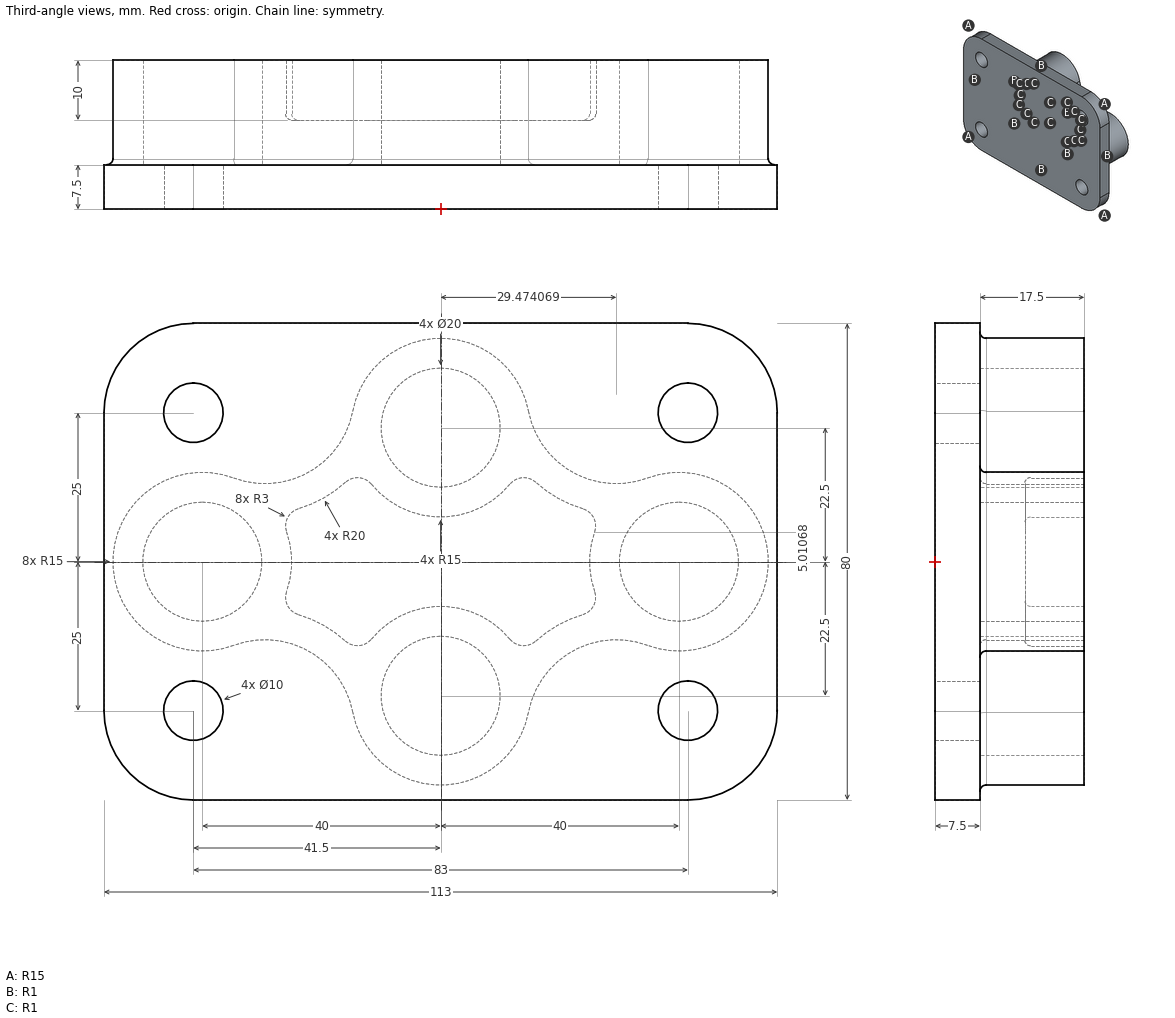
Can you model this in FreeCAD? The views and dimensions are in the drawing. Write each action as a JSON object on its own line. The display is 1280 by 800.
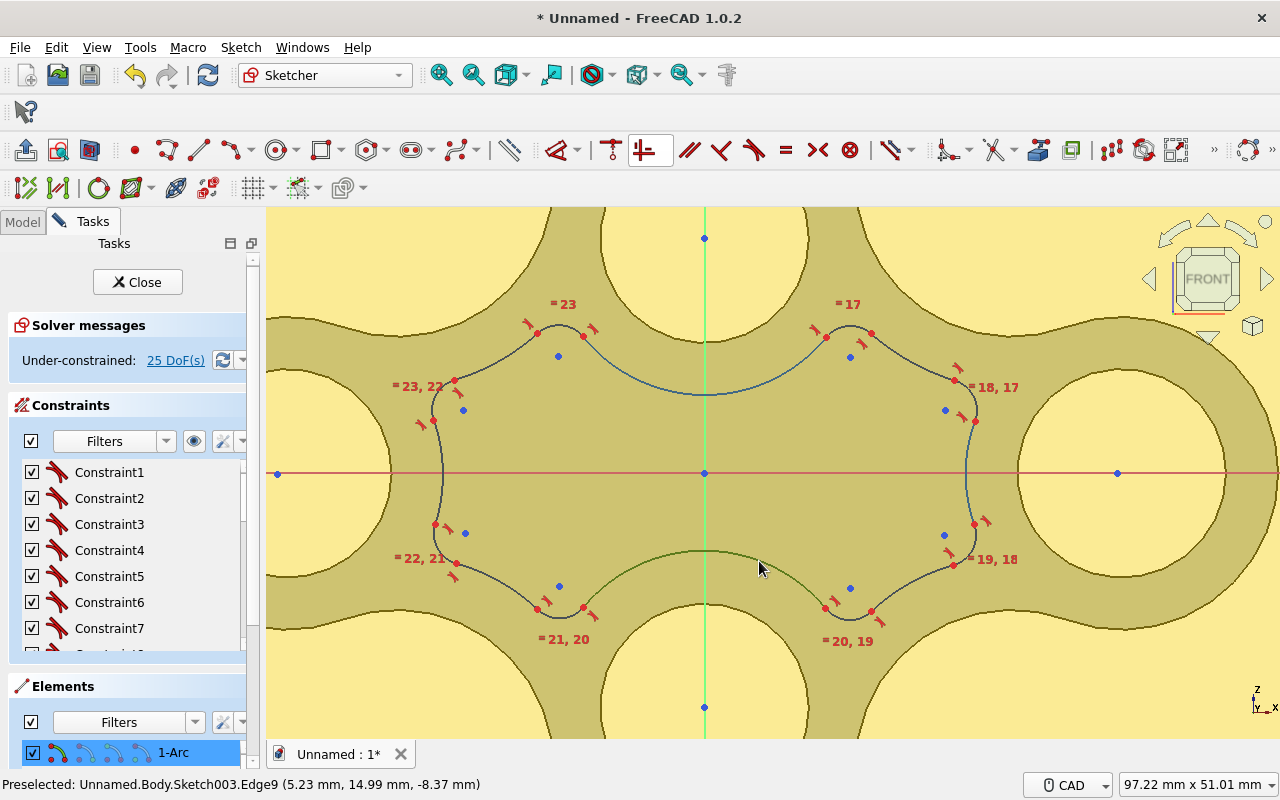
{"action": "left_click", "coordinate": [442, 493]}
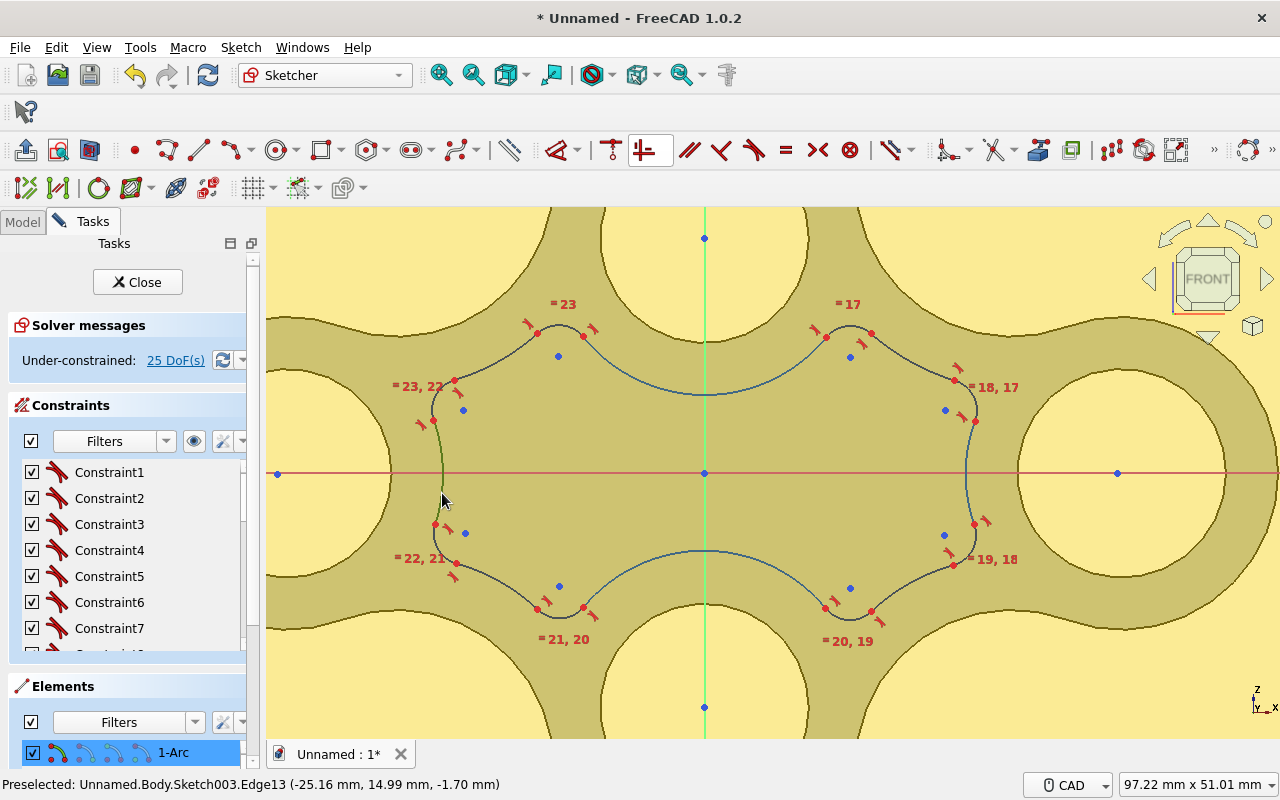
{"action": "key", "text": "e"}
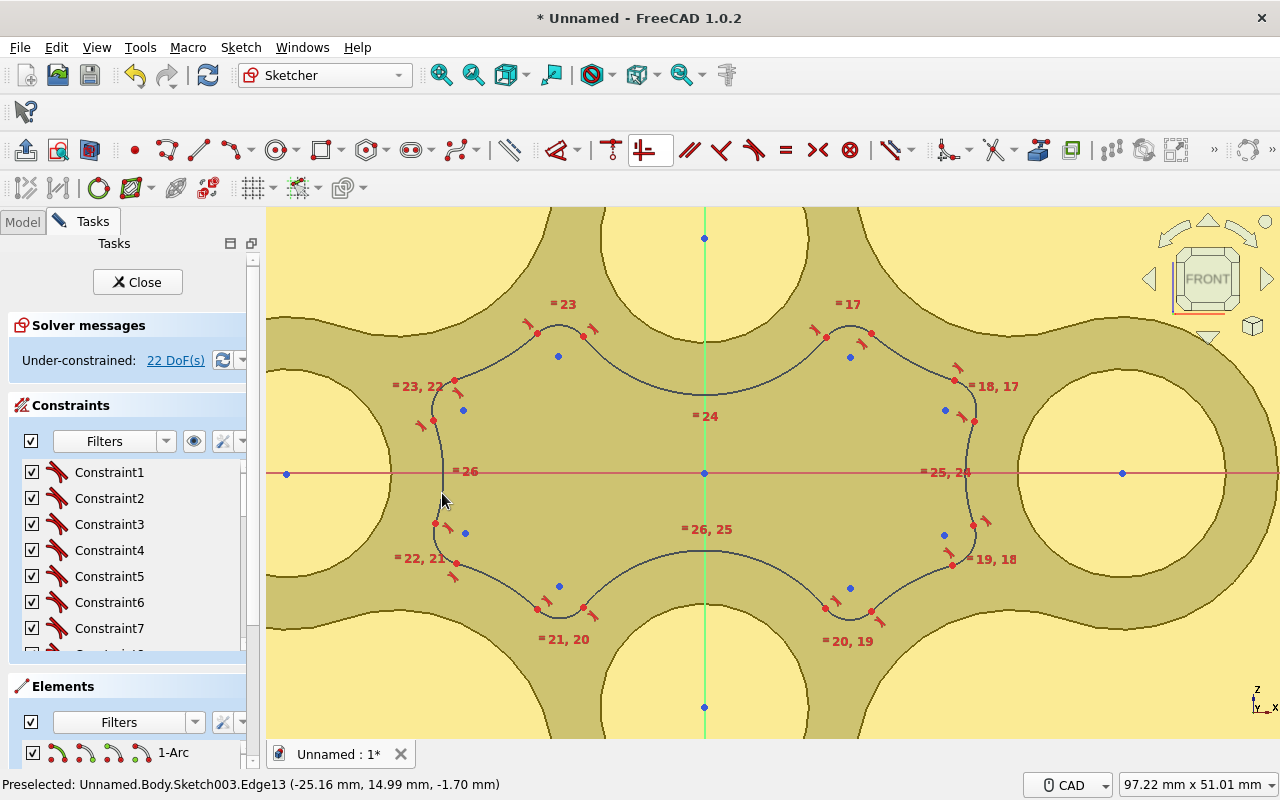
{"action": "left_click", "coordinate": [894, 351]}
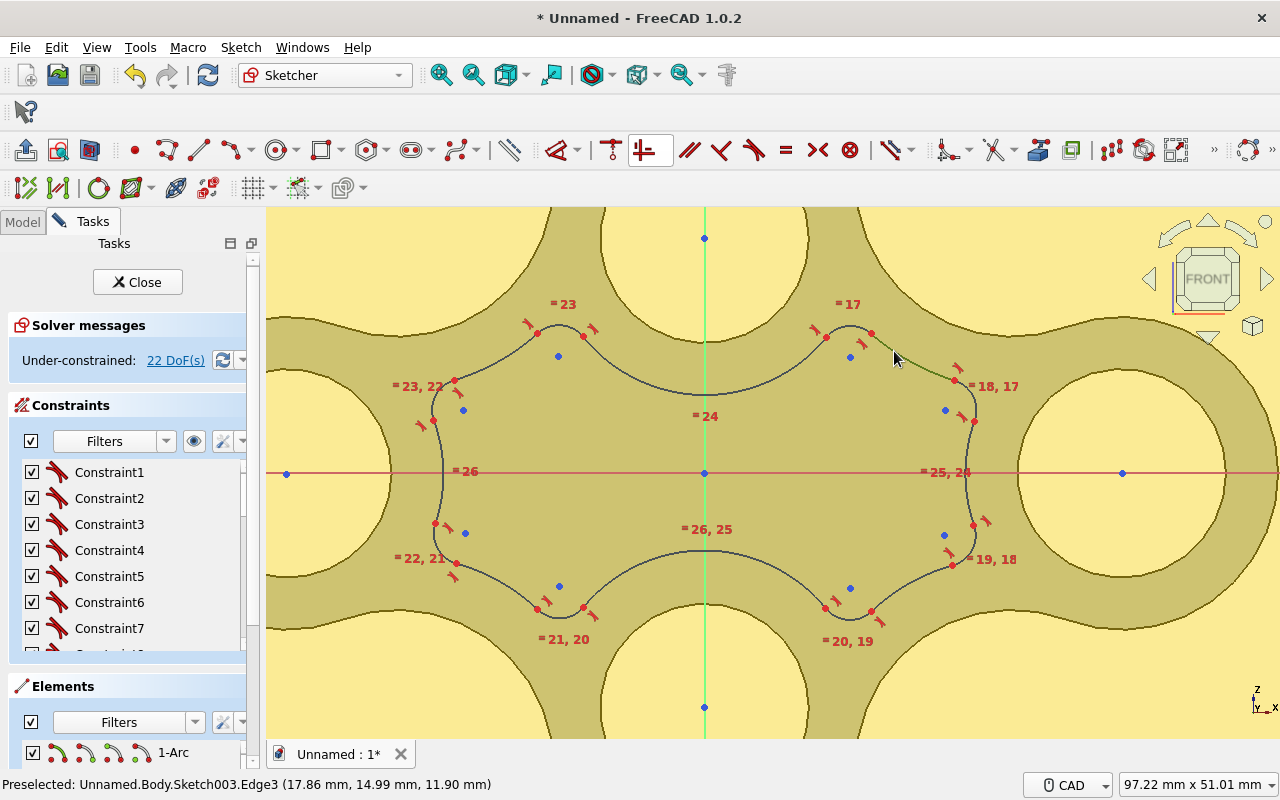
{"action": "left_click", "coordinate": [926, 575]}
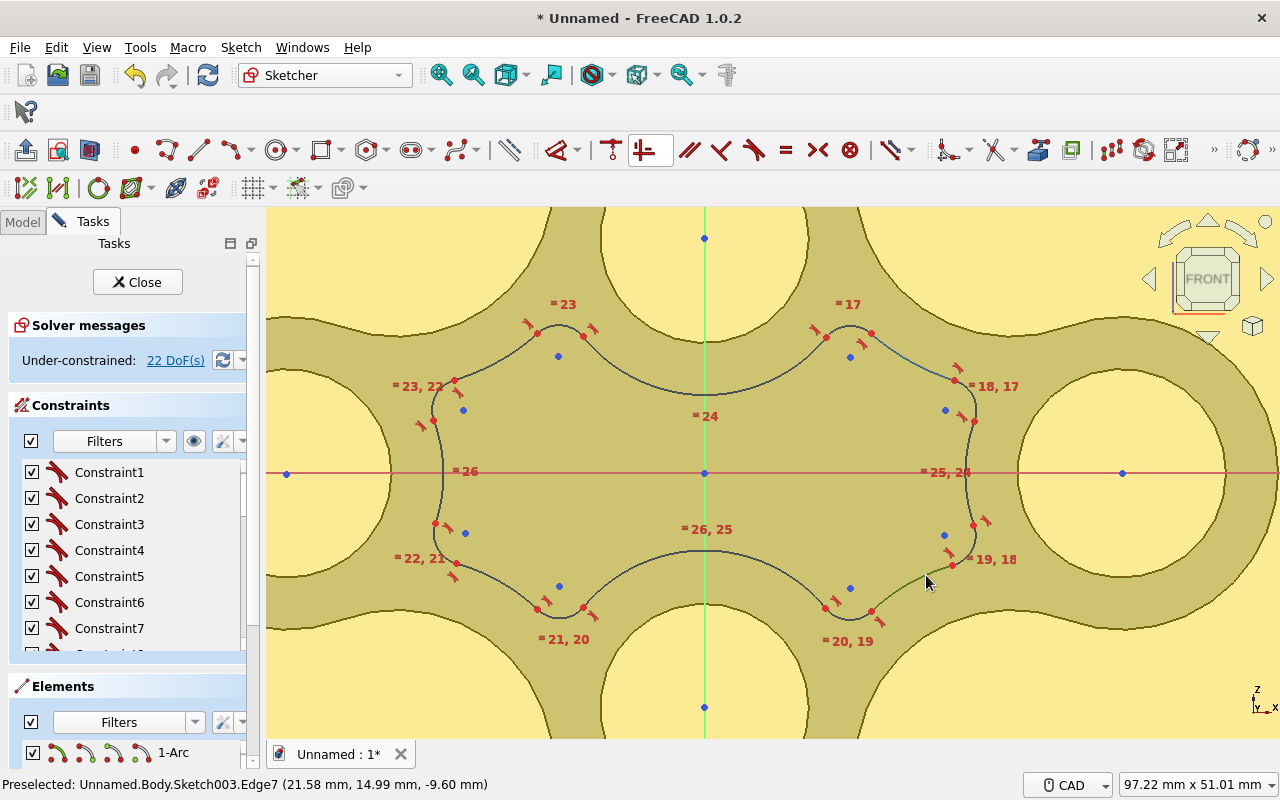
{"action": "left_click", "coordinate": [516, 592]}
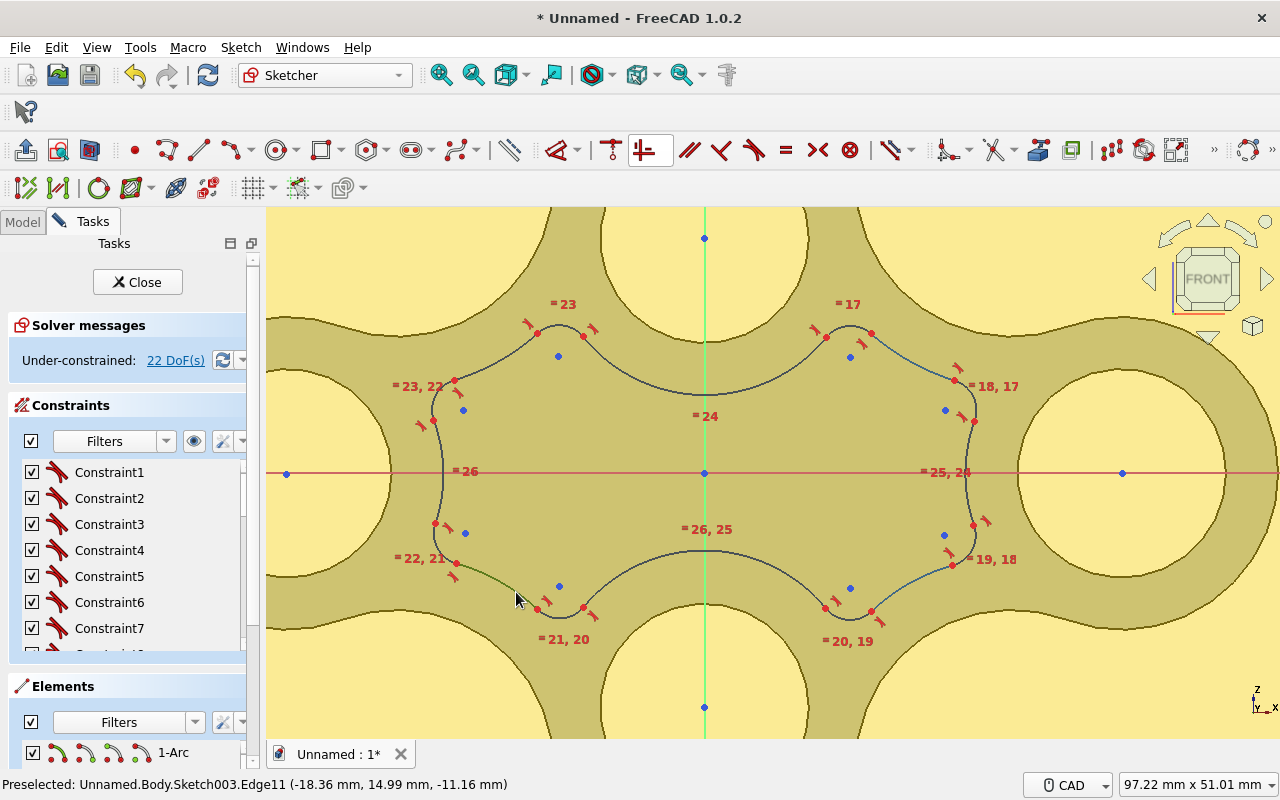
{"action": "left_click", "coordinate": [482, 370]}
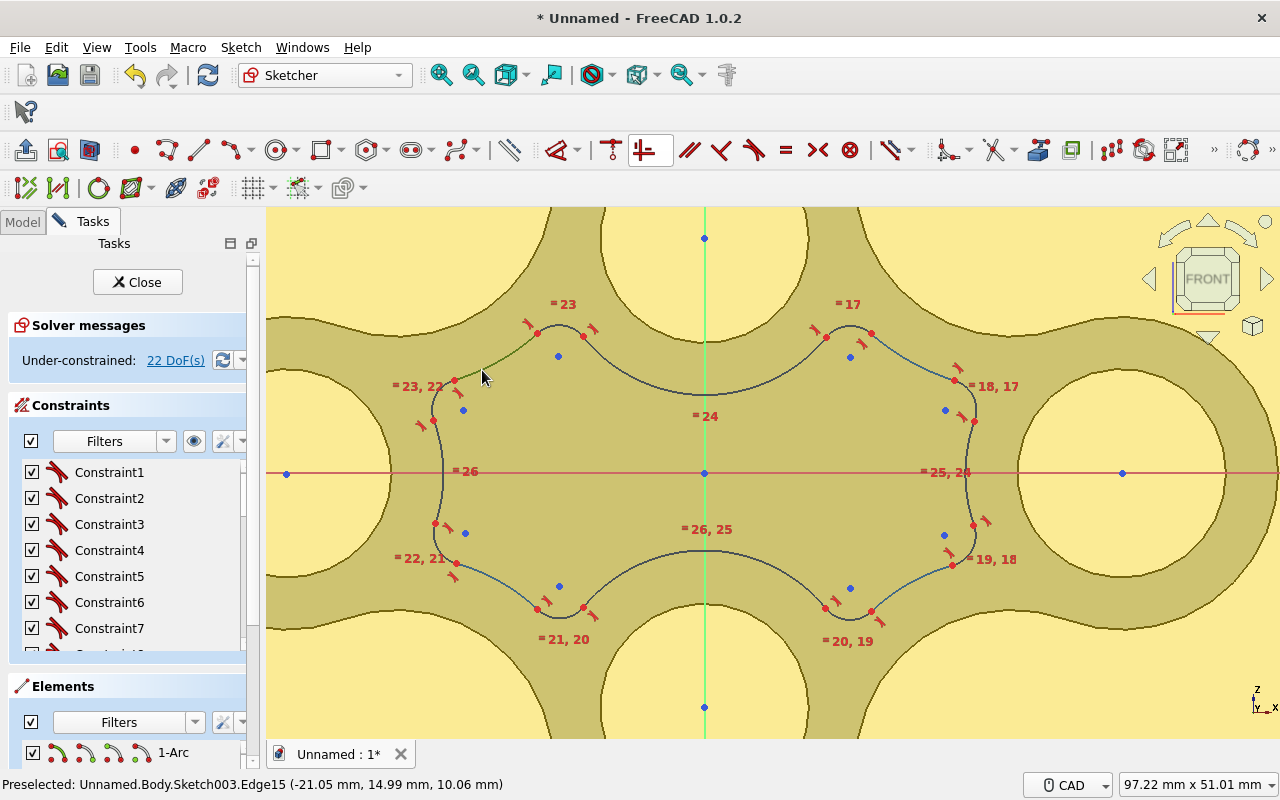
{"action": "key", "text": "e"}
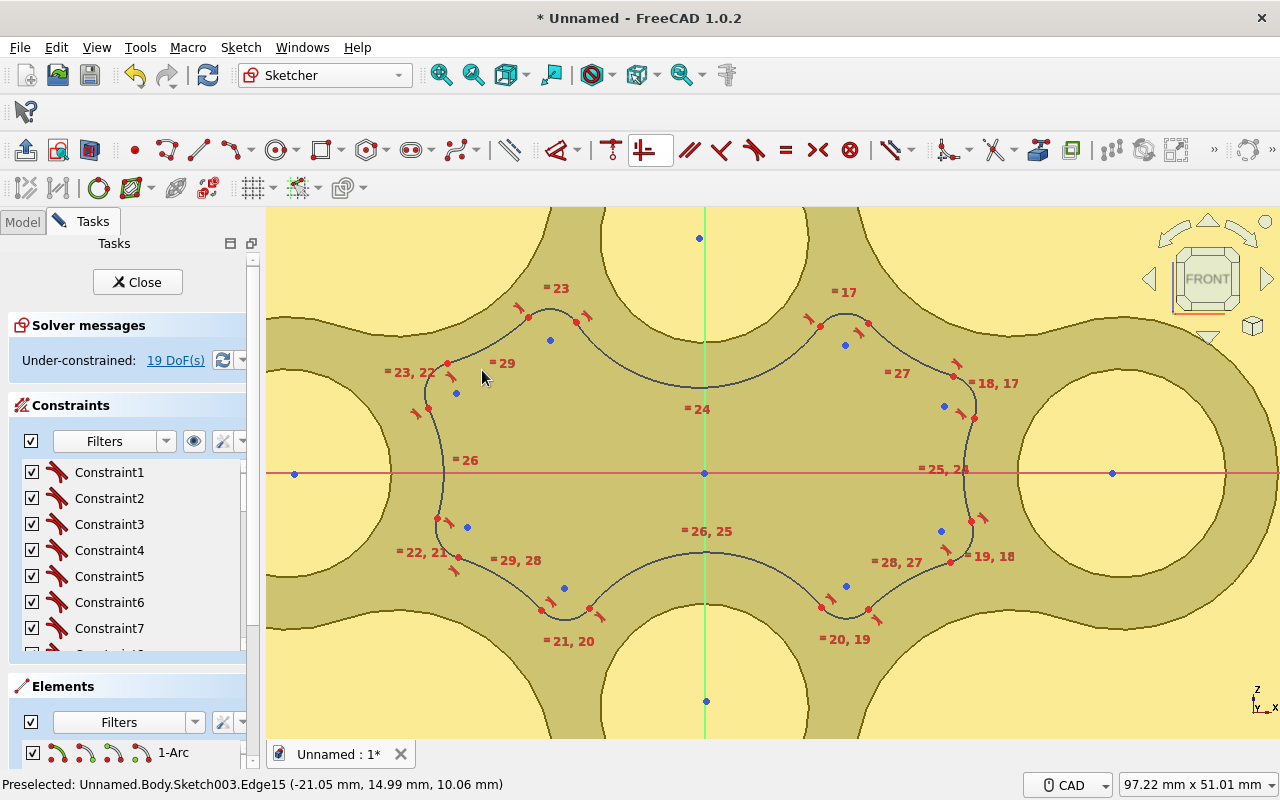
{"action": "left_click", "coordinate": [699, 238]}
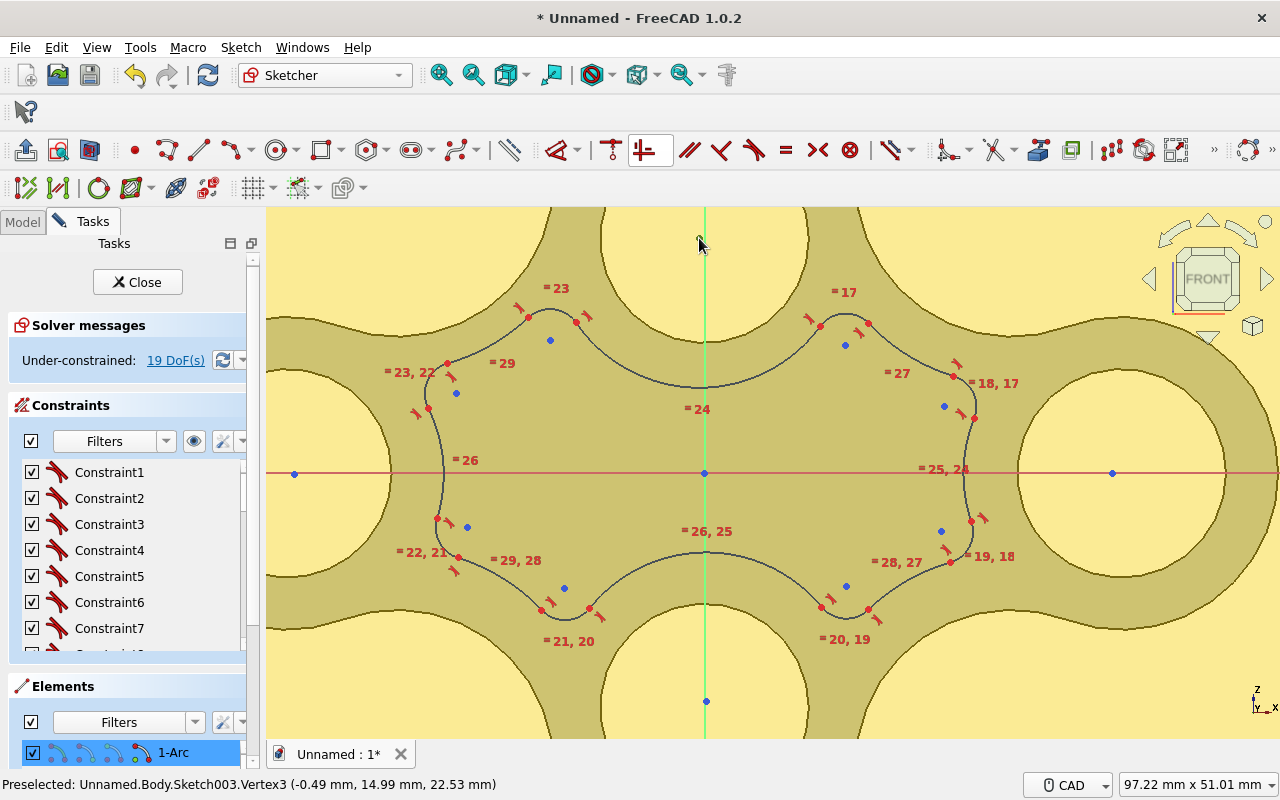
{"action": "left_click", "coordinate": [705, 677]}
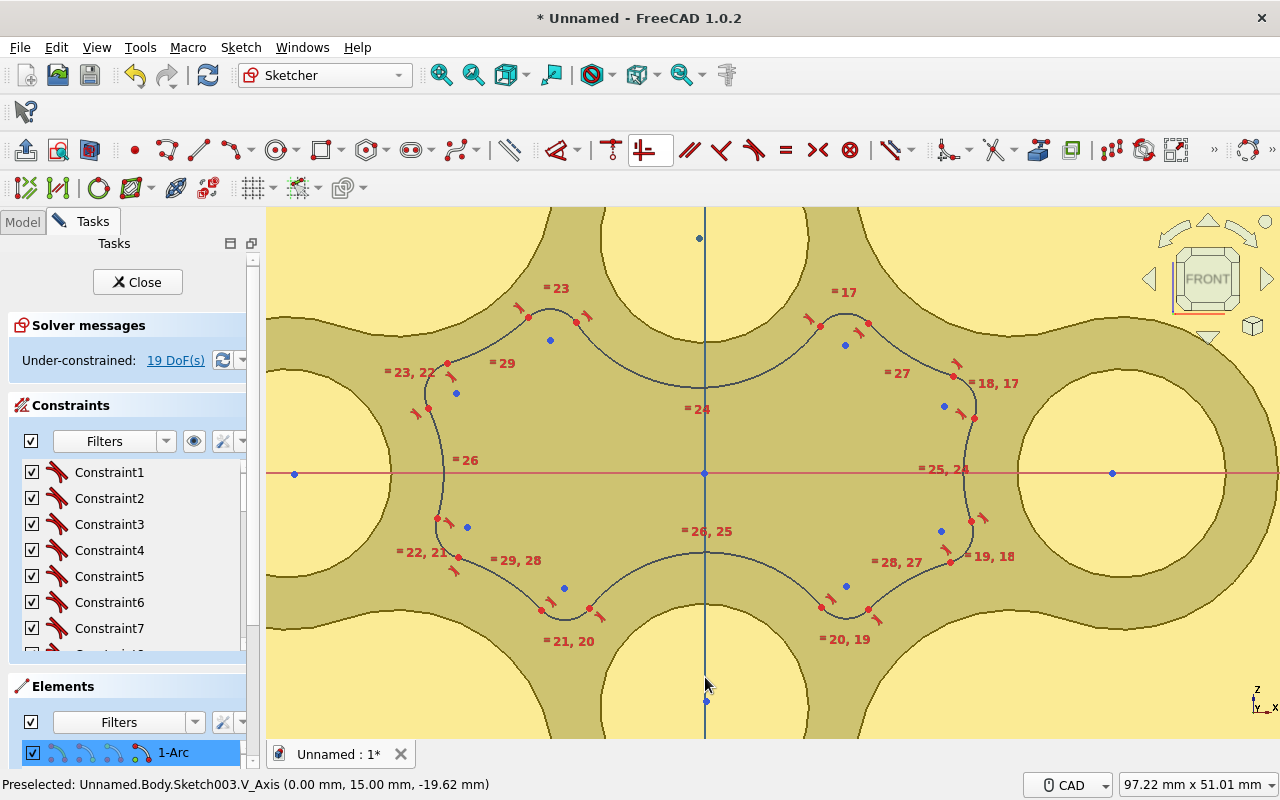
{"action": "left_click", "coordinate": [612, 150]}